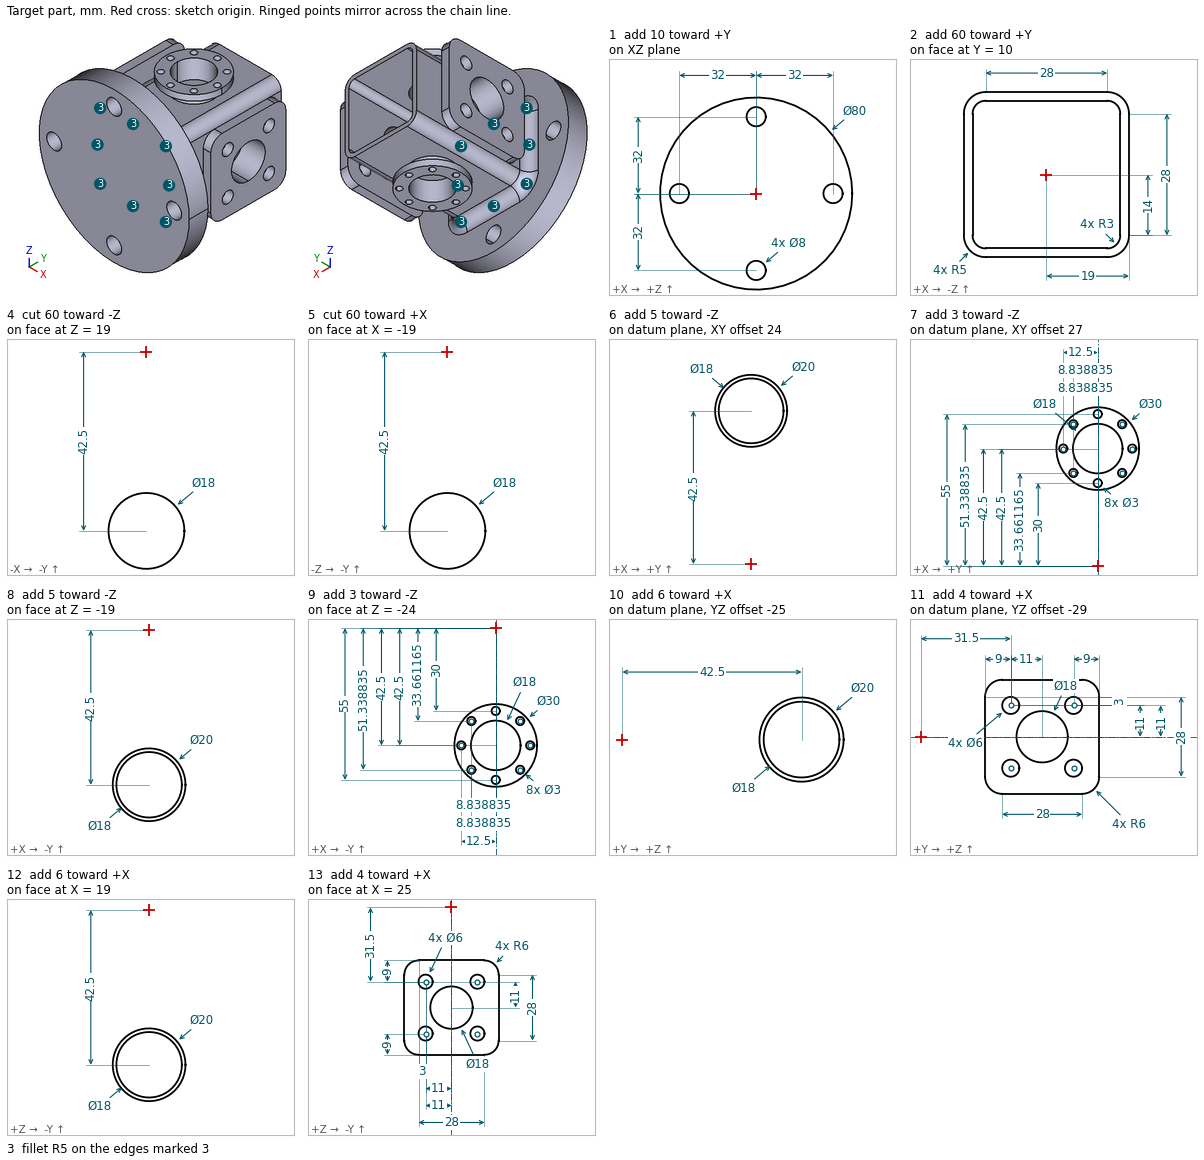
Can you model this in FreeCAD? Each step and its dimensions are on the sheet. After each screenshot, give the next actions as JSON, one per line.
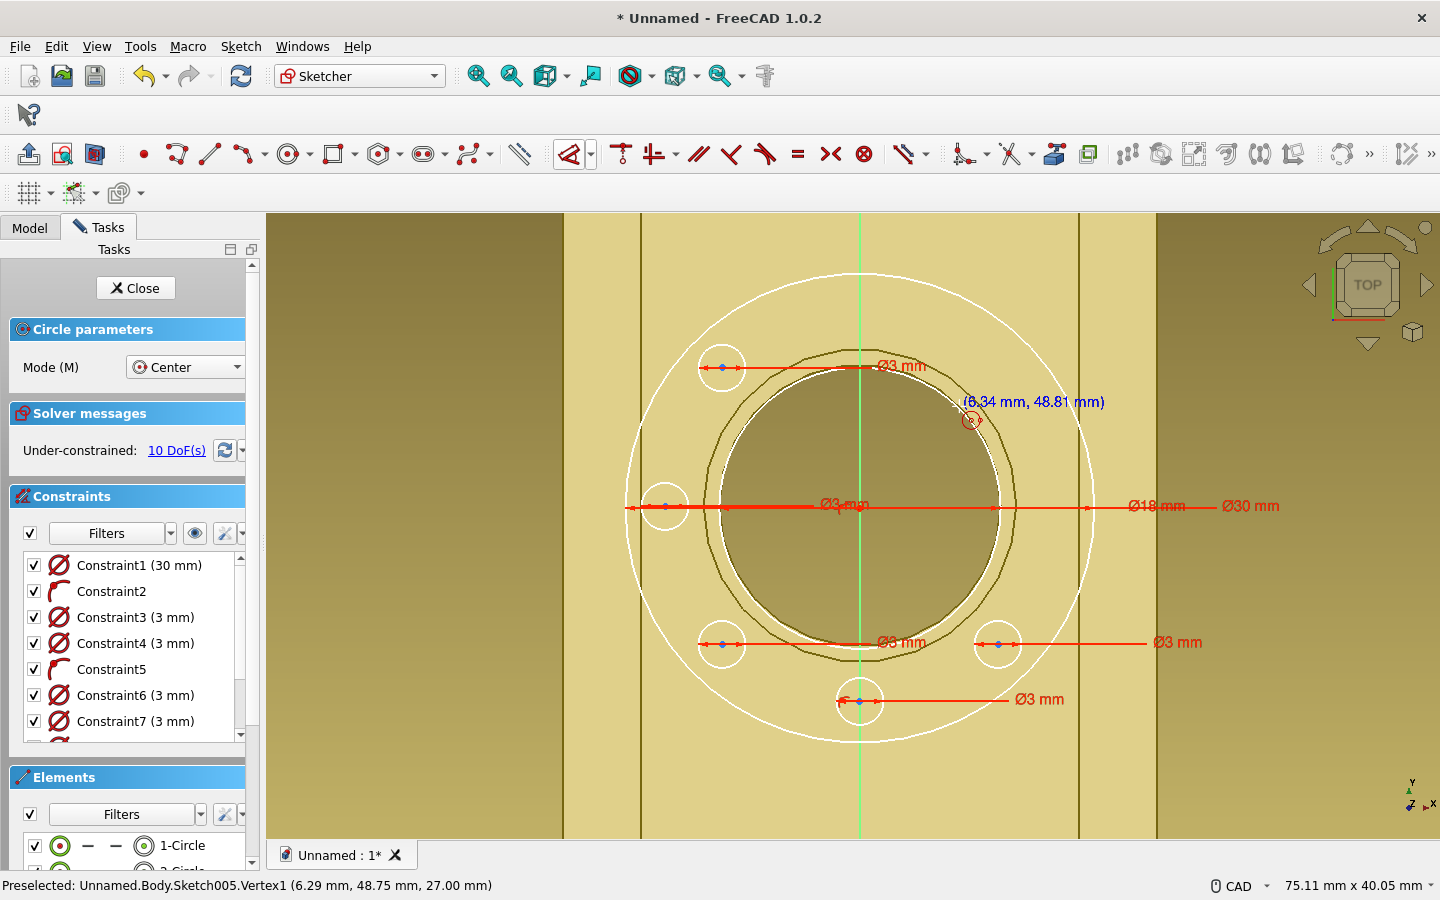
{"action": "left_click", "coordinate": [1055, 506]}
{"action": "mouse_move", "coordinate": [1072, 489]}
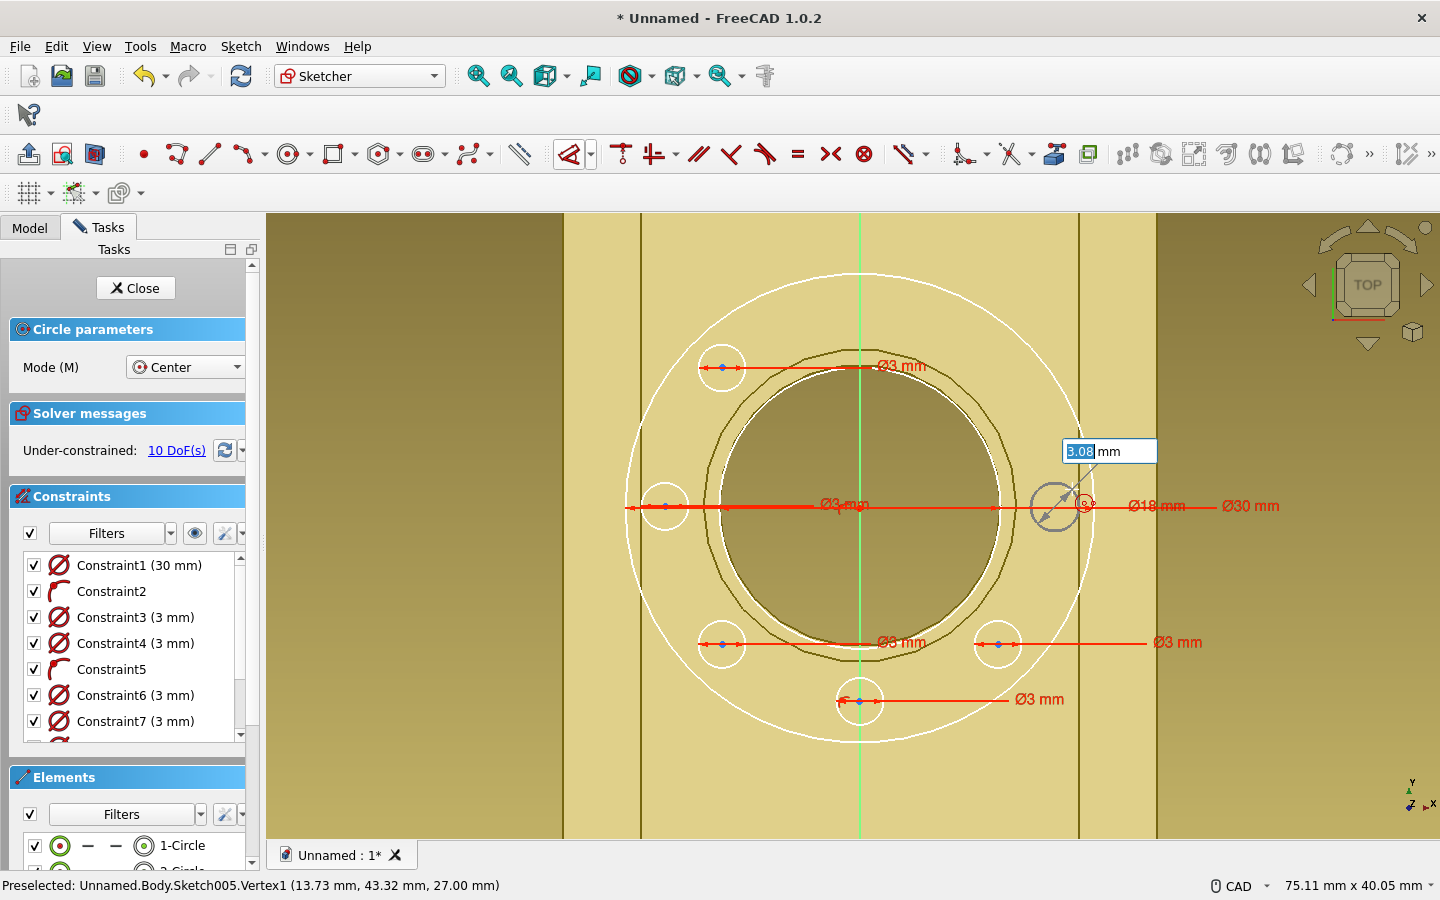
{"action": "type", "text": "3"}
{"action": "key", "text": "Return"}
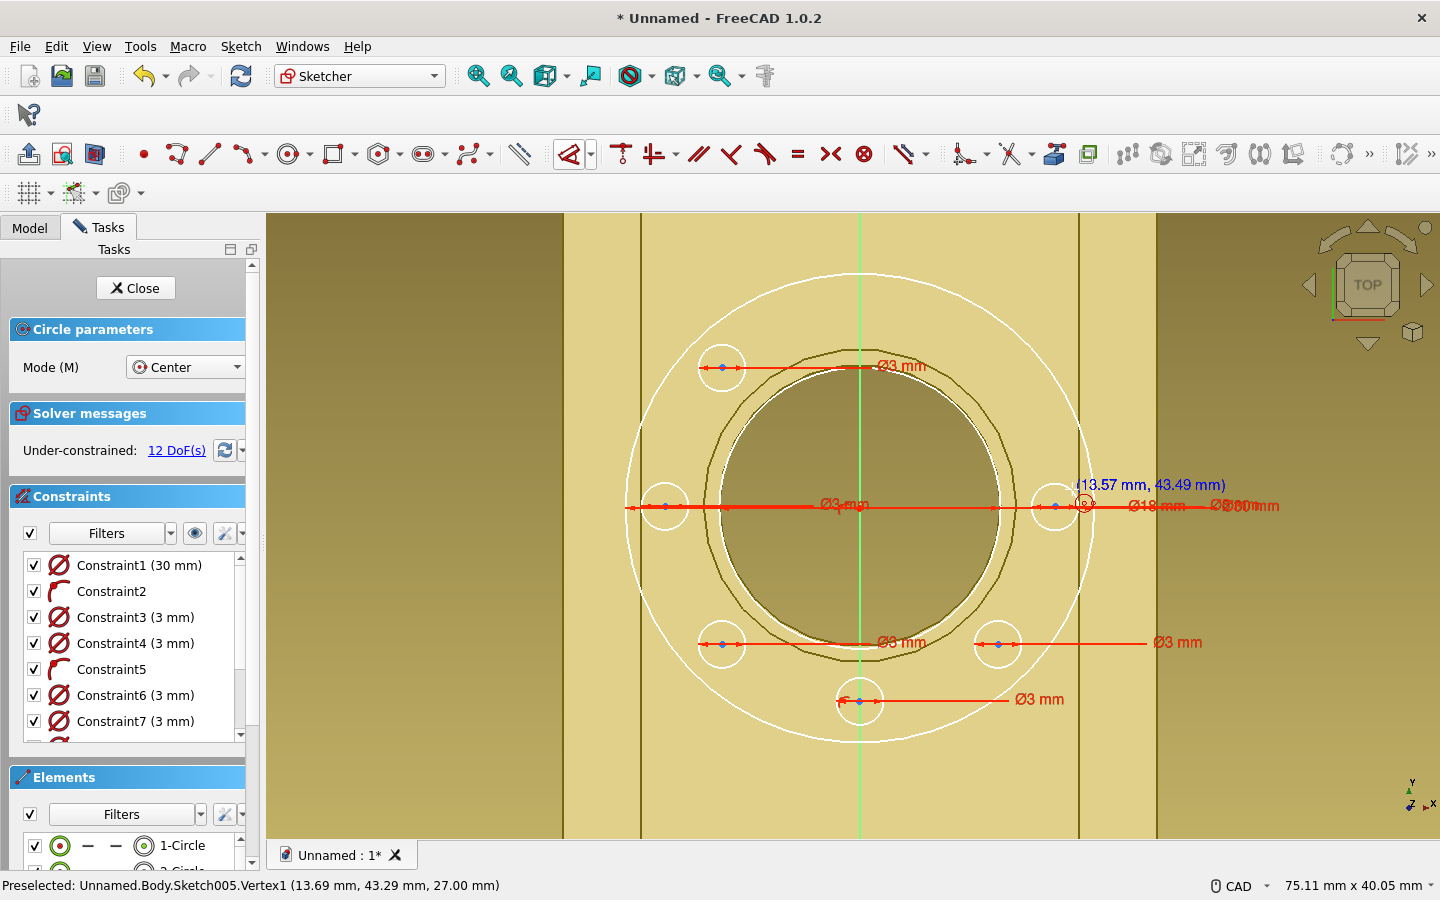
{"action": "left_click", "coordinate": [860, 310]}
{"action": "mouse_move", "coordinate": [877, 294]}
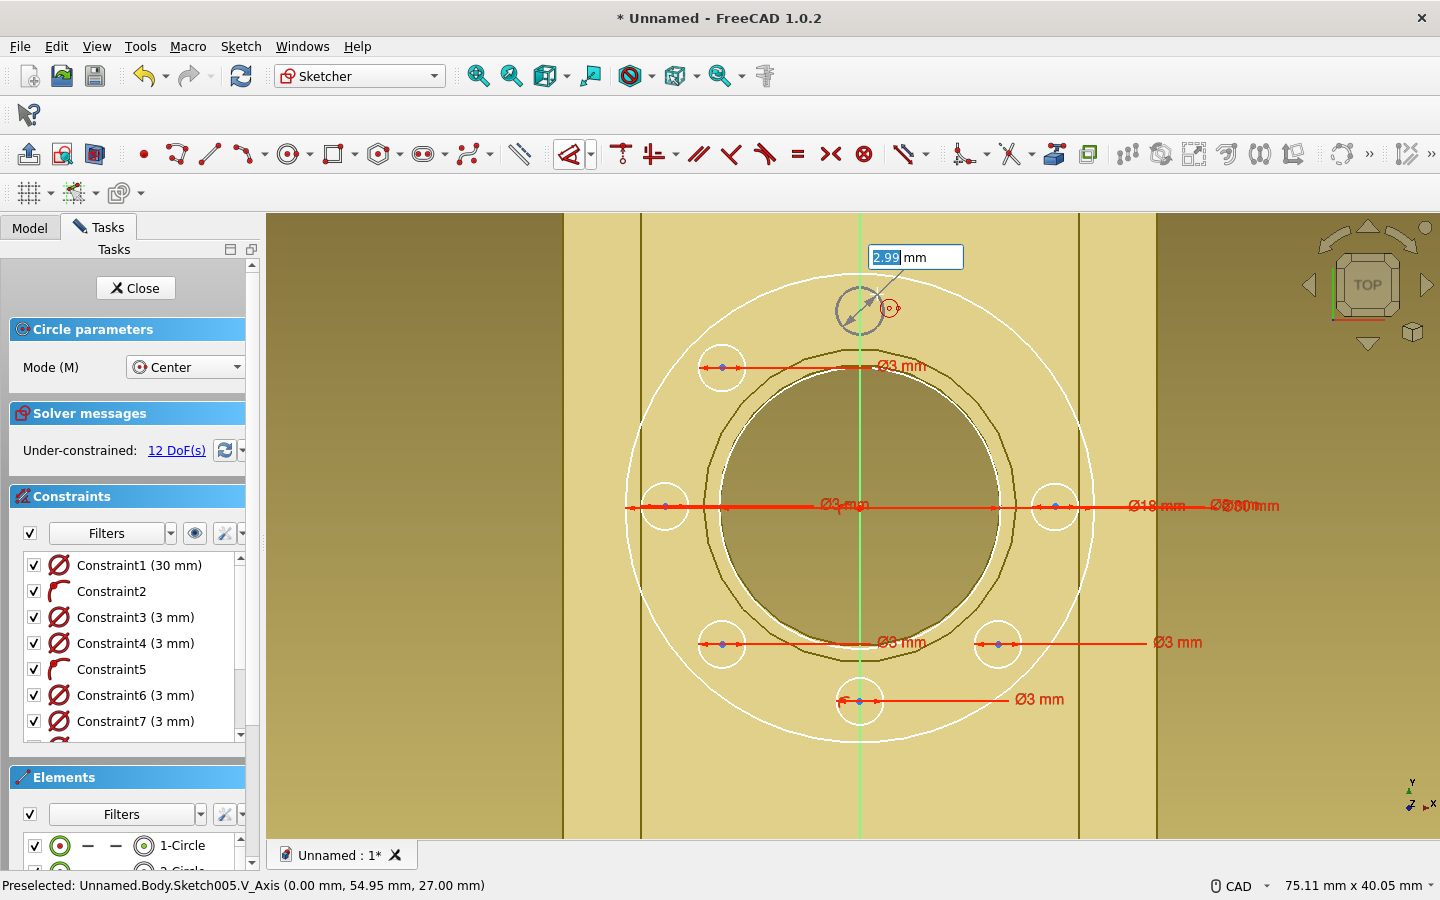
{"action": "type", "text": "3"}
{"action": "key", "text": "Return"}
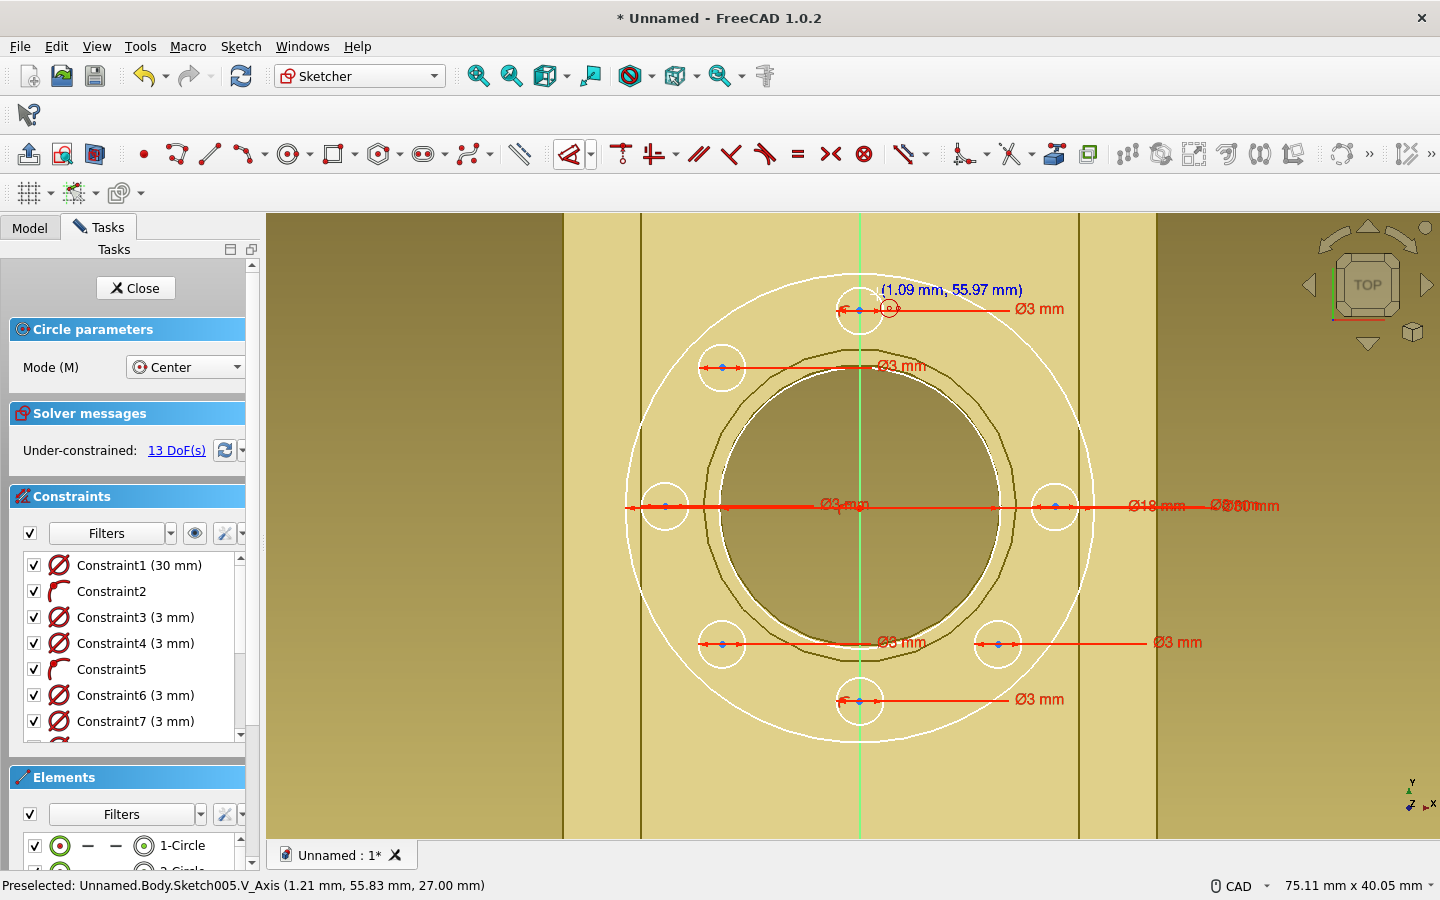
{"action": "left_click", "coordinate": [998, 367]}
{"action": "mouse_move", "coordinate": [1015, 351]}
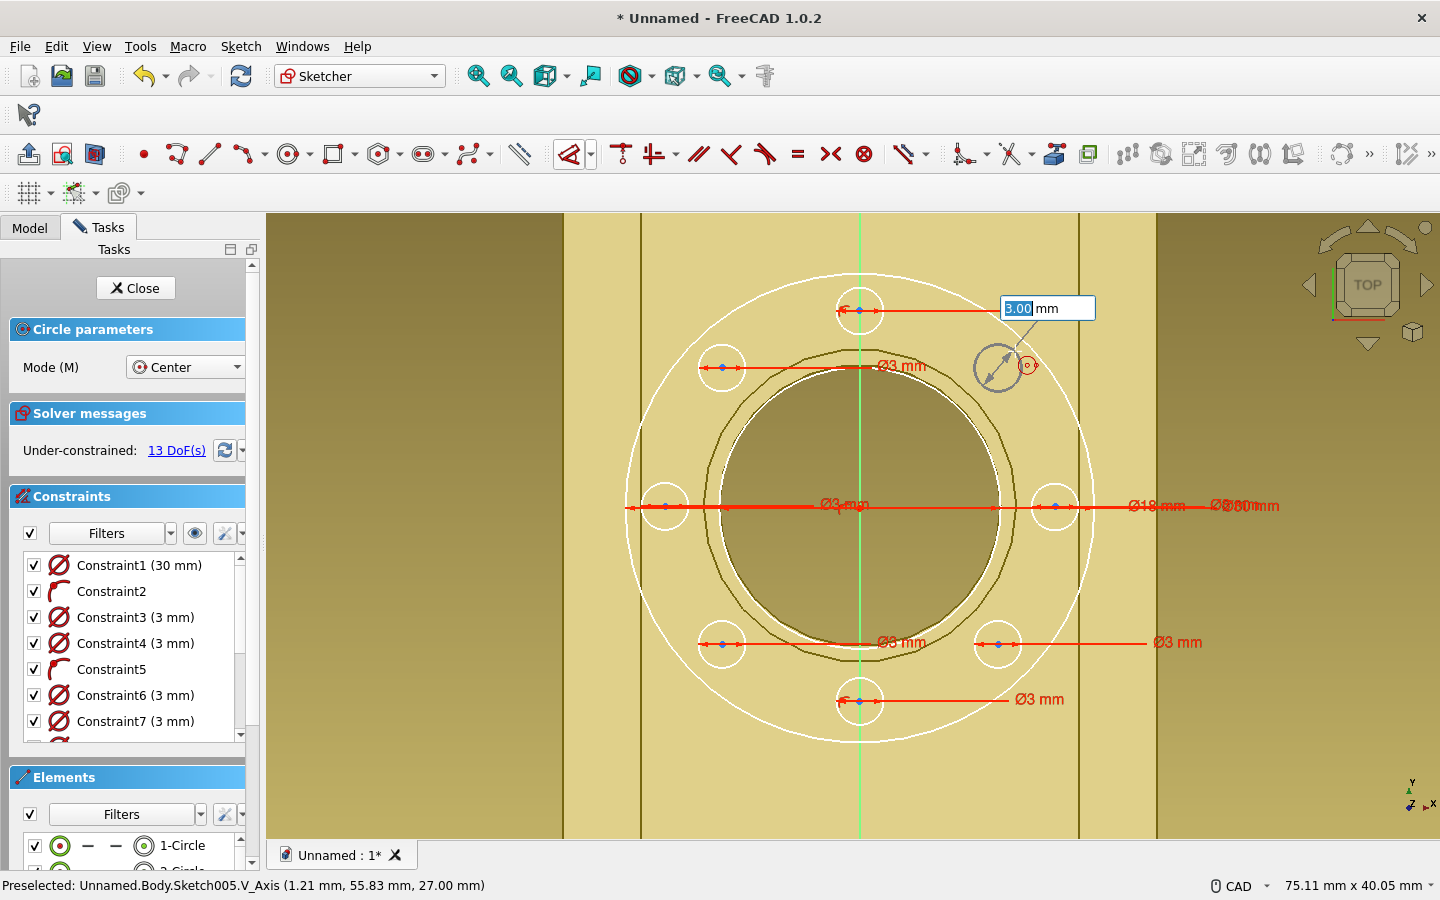
{"action": "type", "text": "3"}
{"action": "key", "text": "Return"}
{"action": "key", "text": "Escape"}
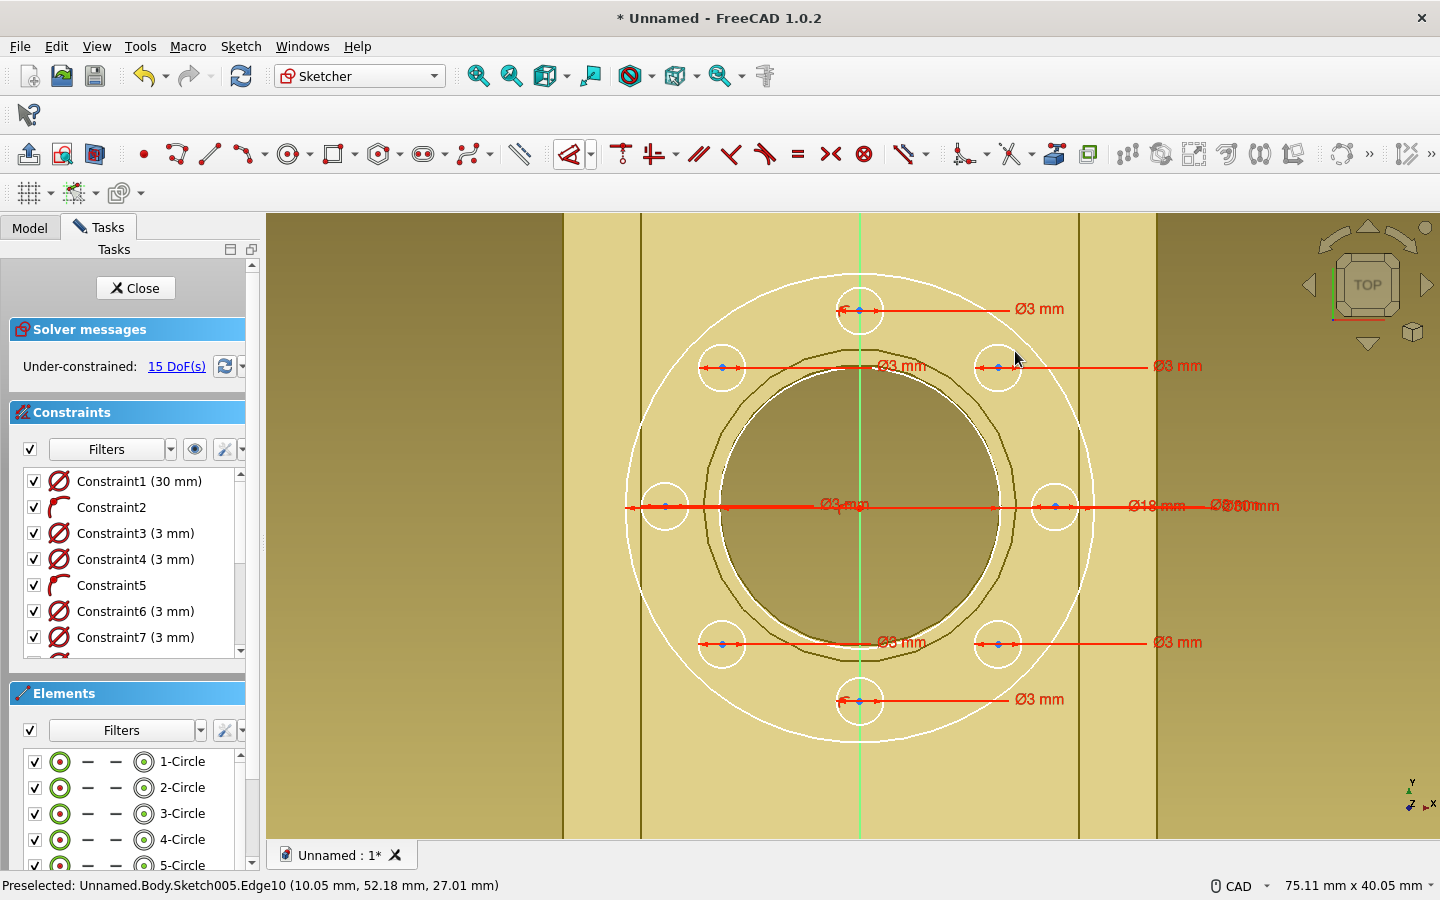
{"action": "left_click", "coordinate": [722, 644]}